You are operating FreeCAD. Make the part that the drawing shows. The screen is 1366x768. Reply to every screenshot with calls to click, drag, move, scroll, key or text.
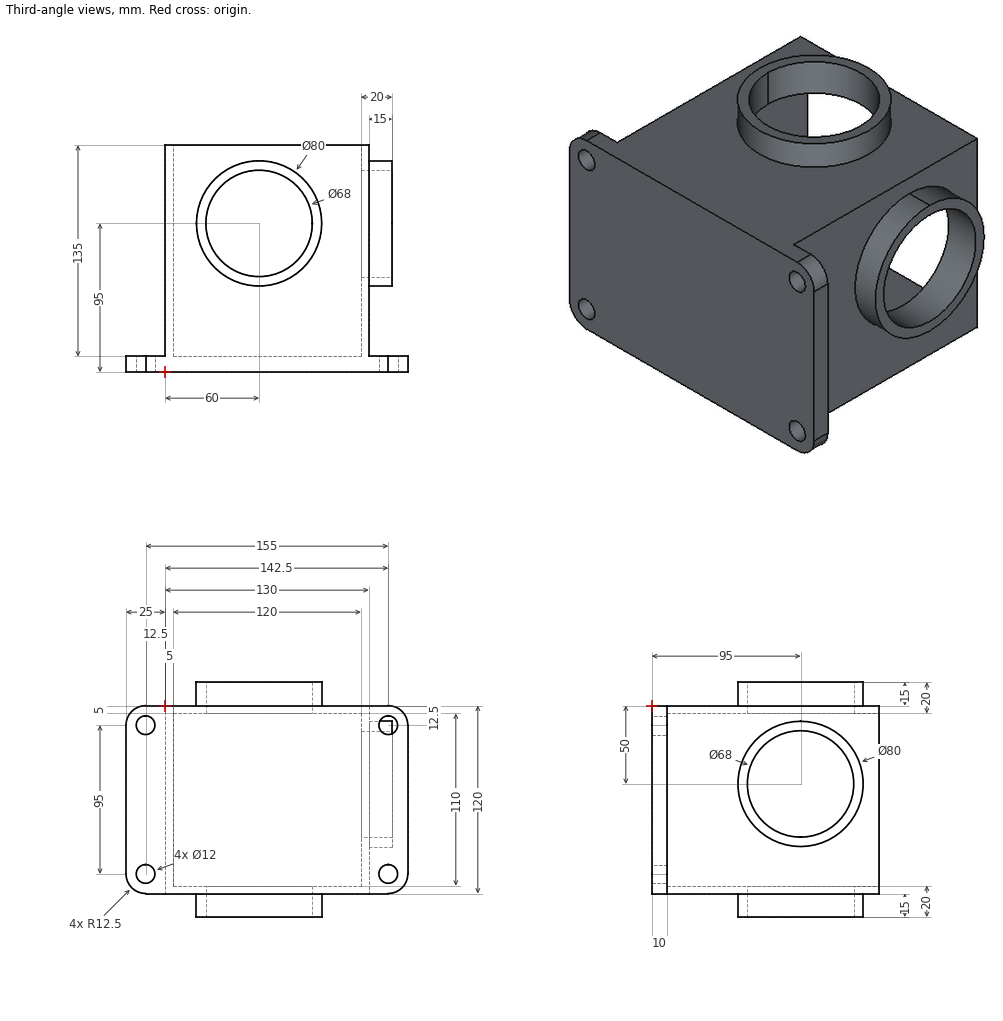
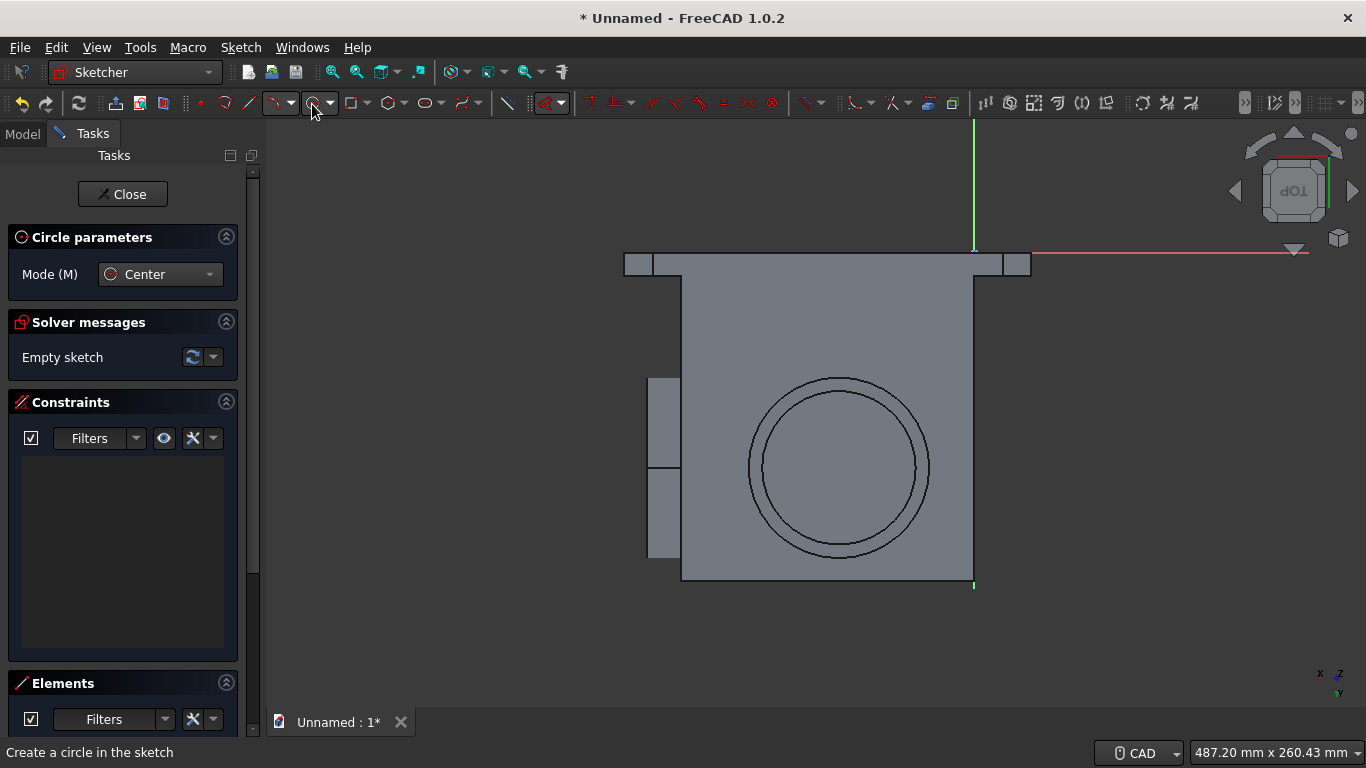
click(839, 468)
move(893, 414)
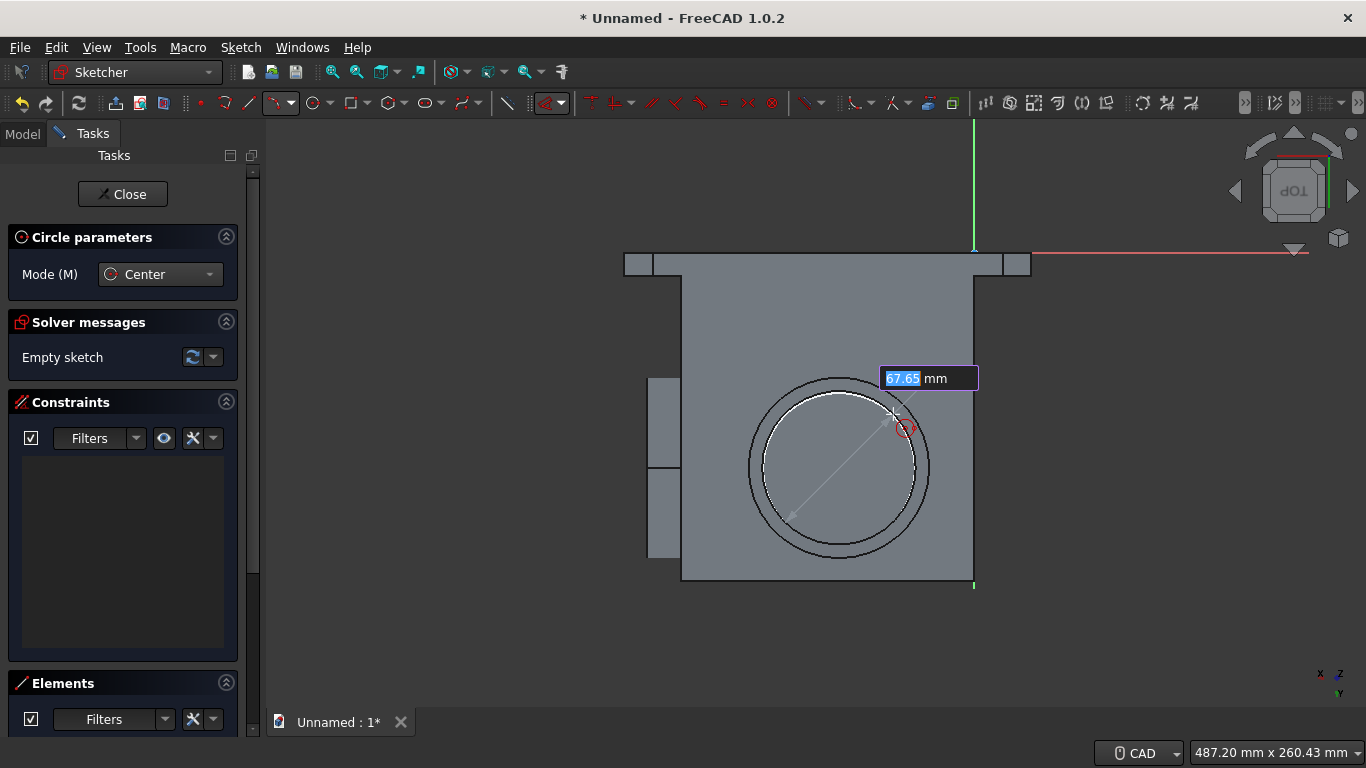
text(68)
key(Return)
key(Escape)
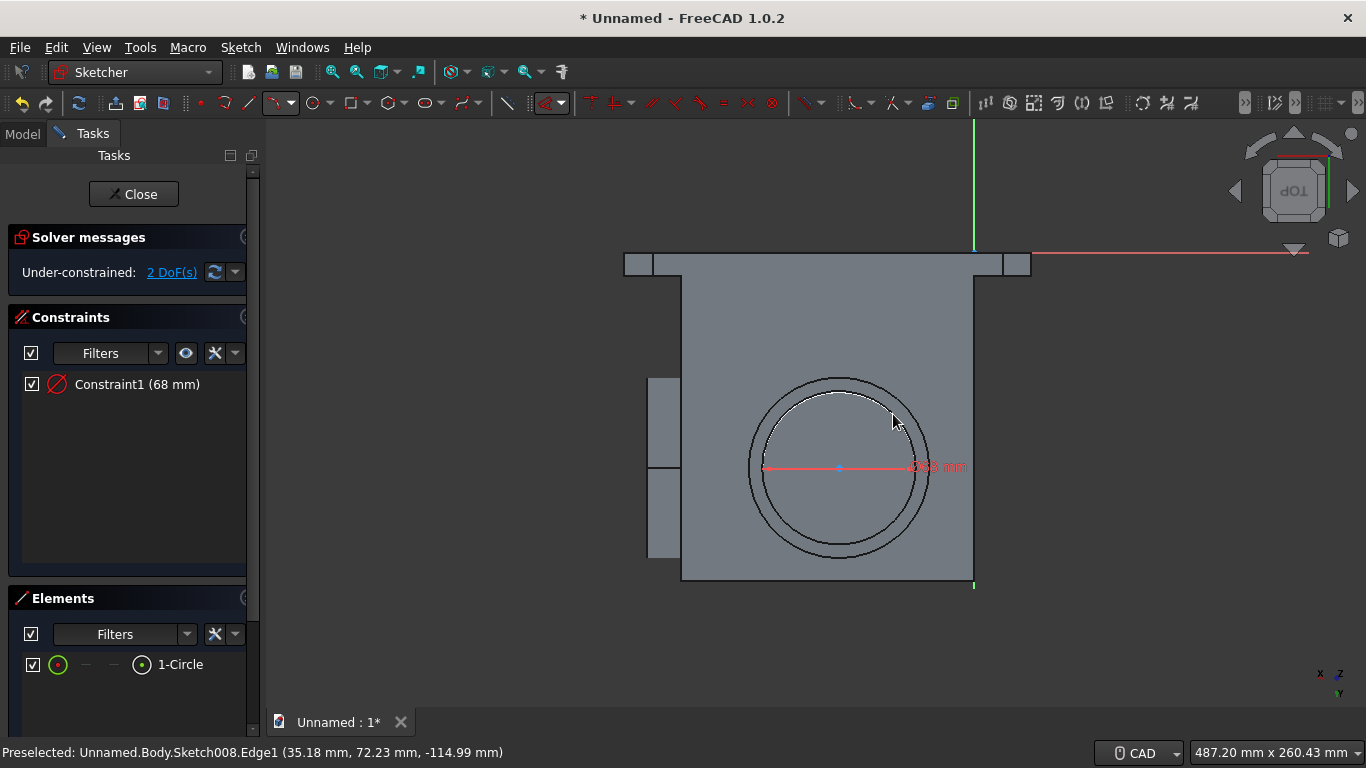
click(839, 469)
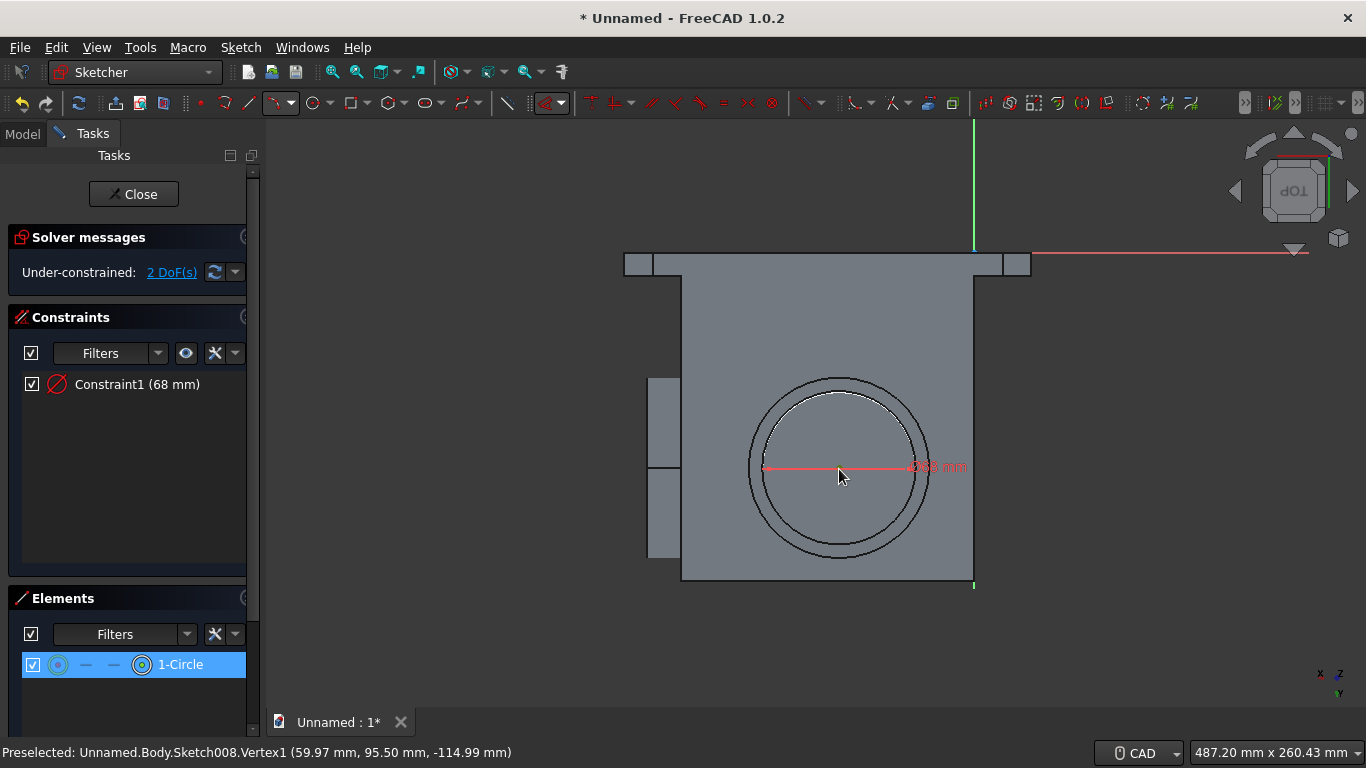
key(l)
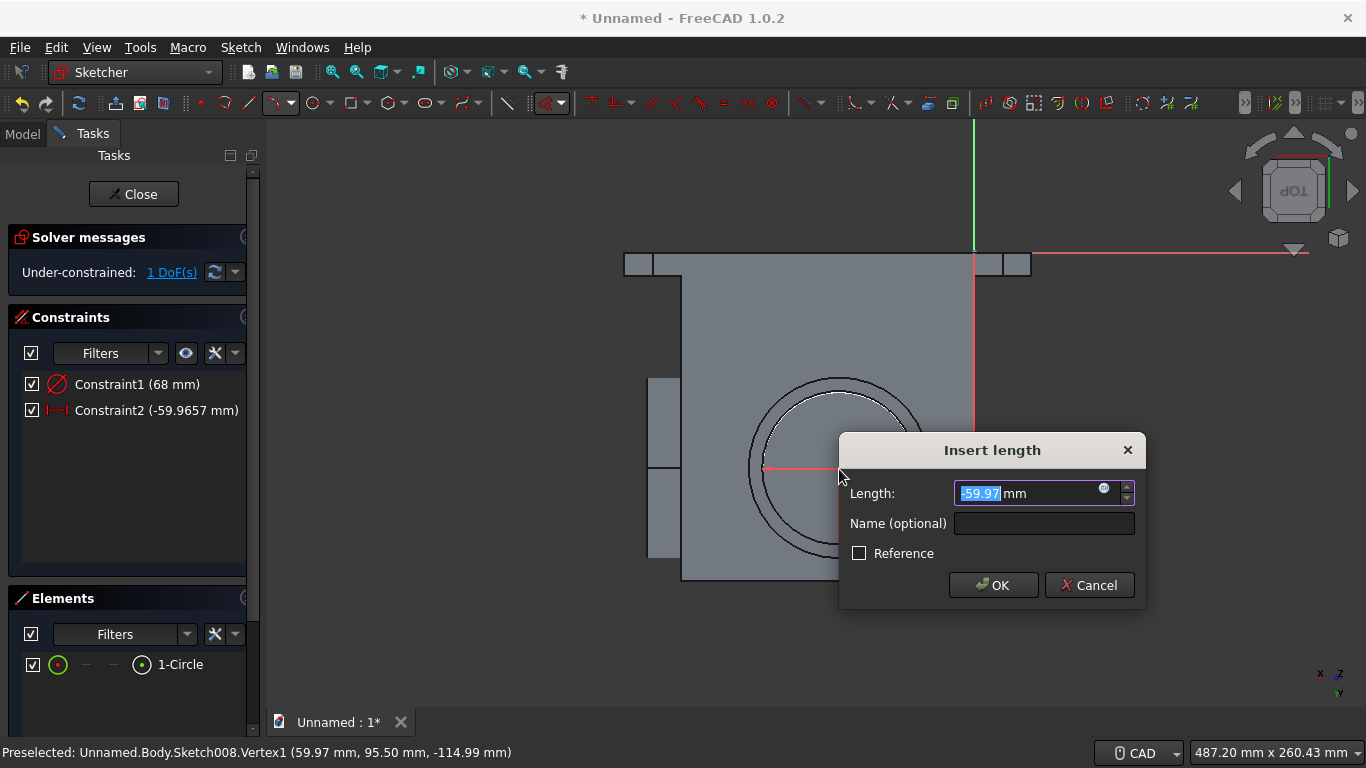
text(-60)
key(Return)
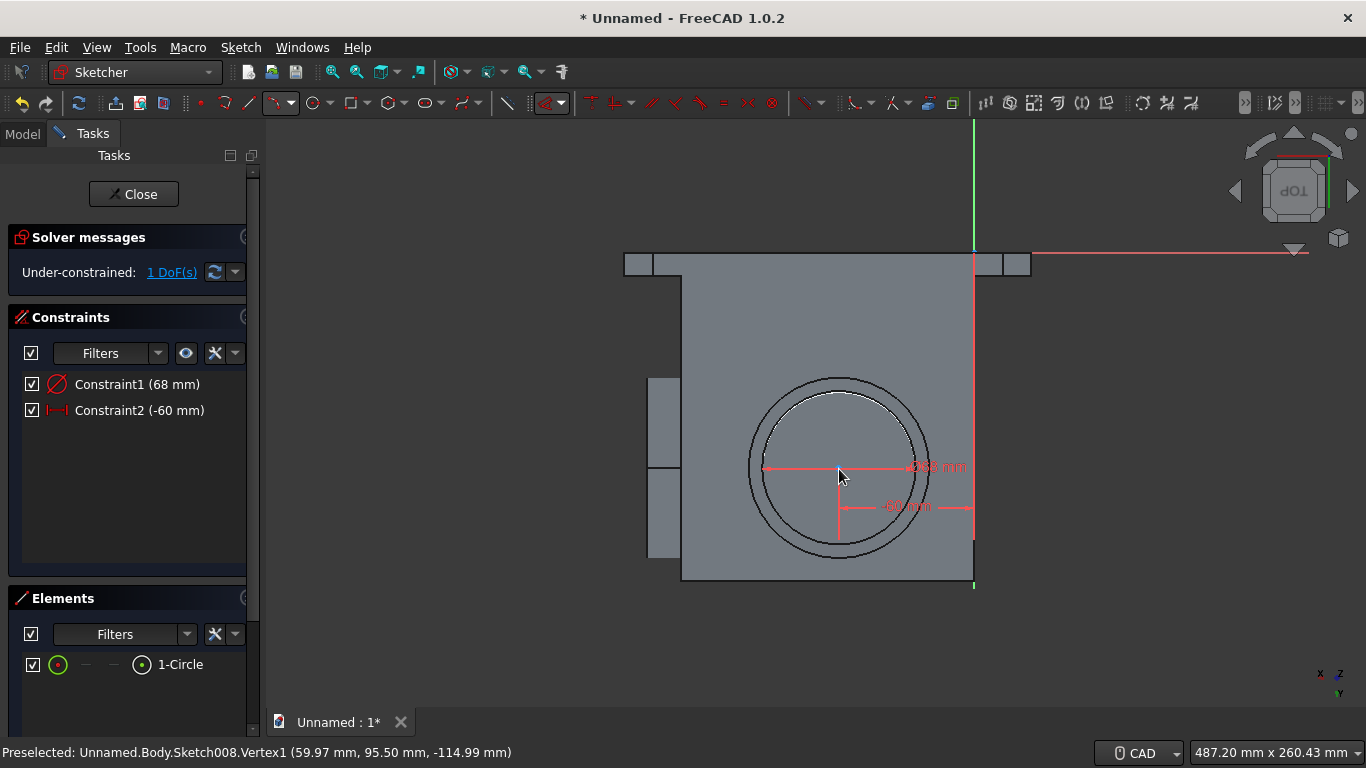
click(839, 469)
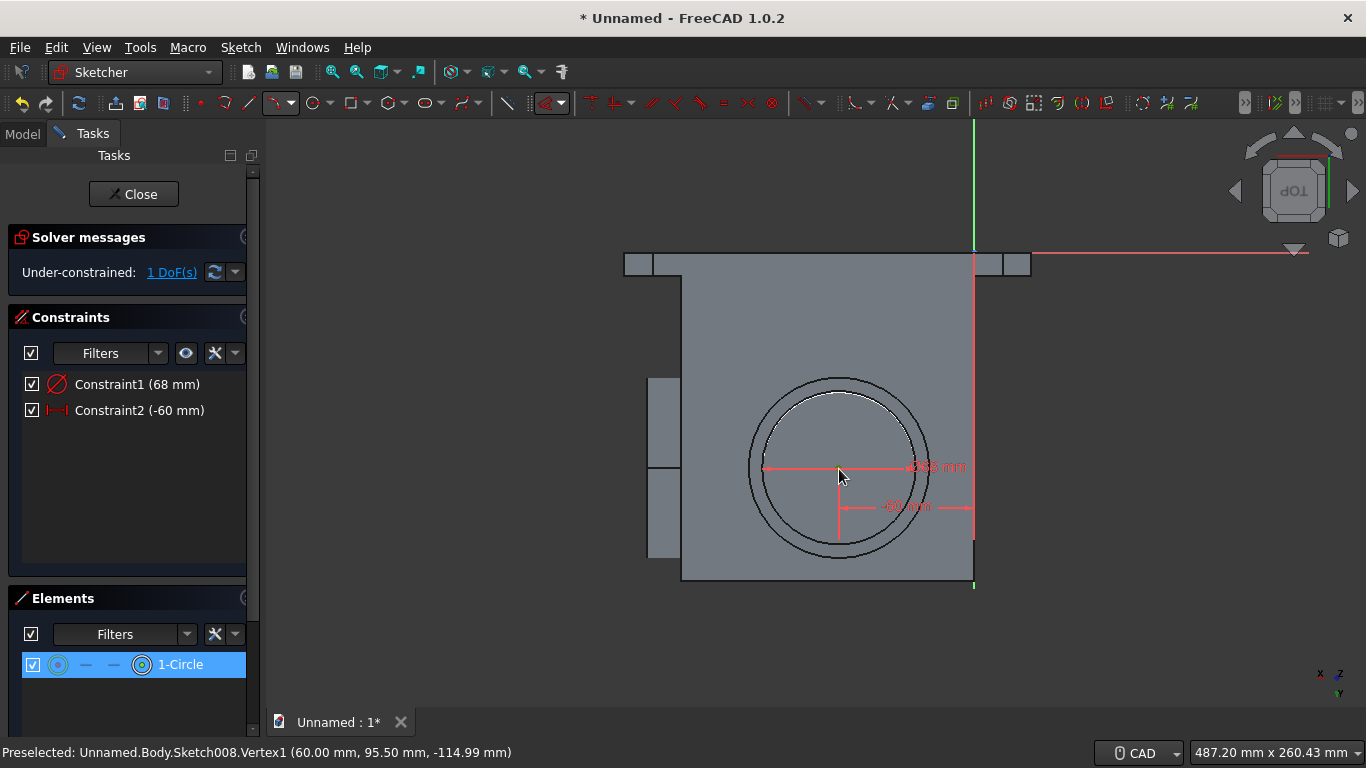
click(564, 104)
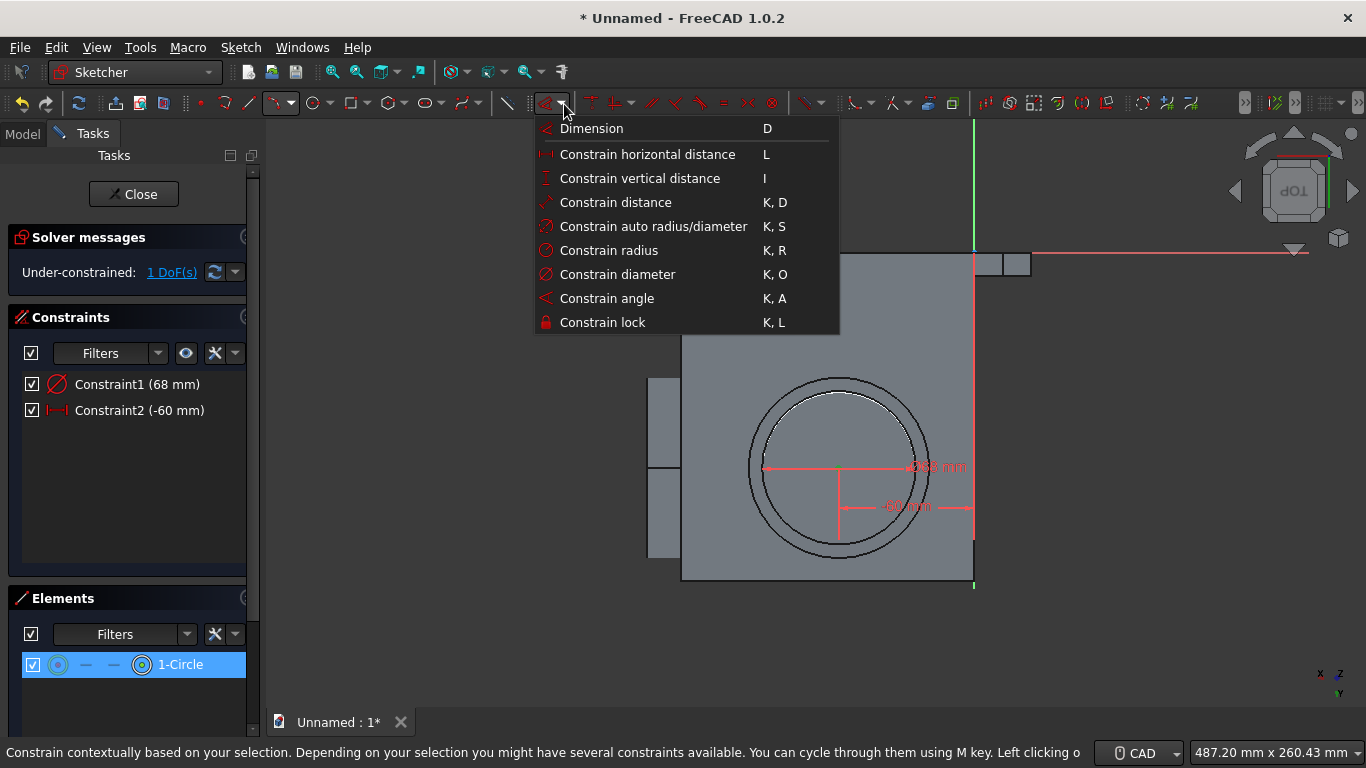
click(687, 178)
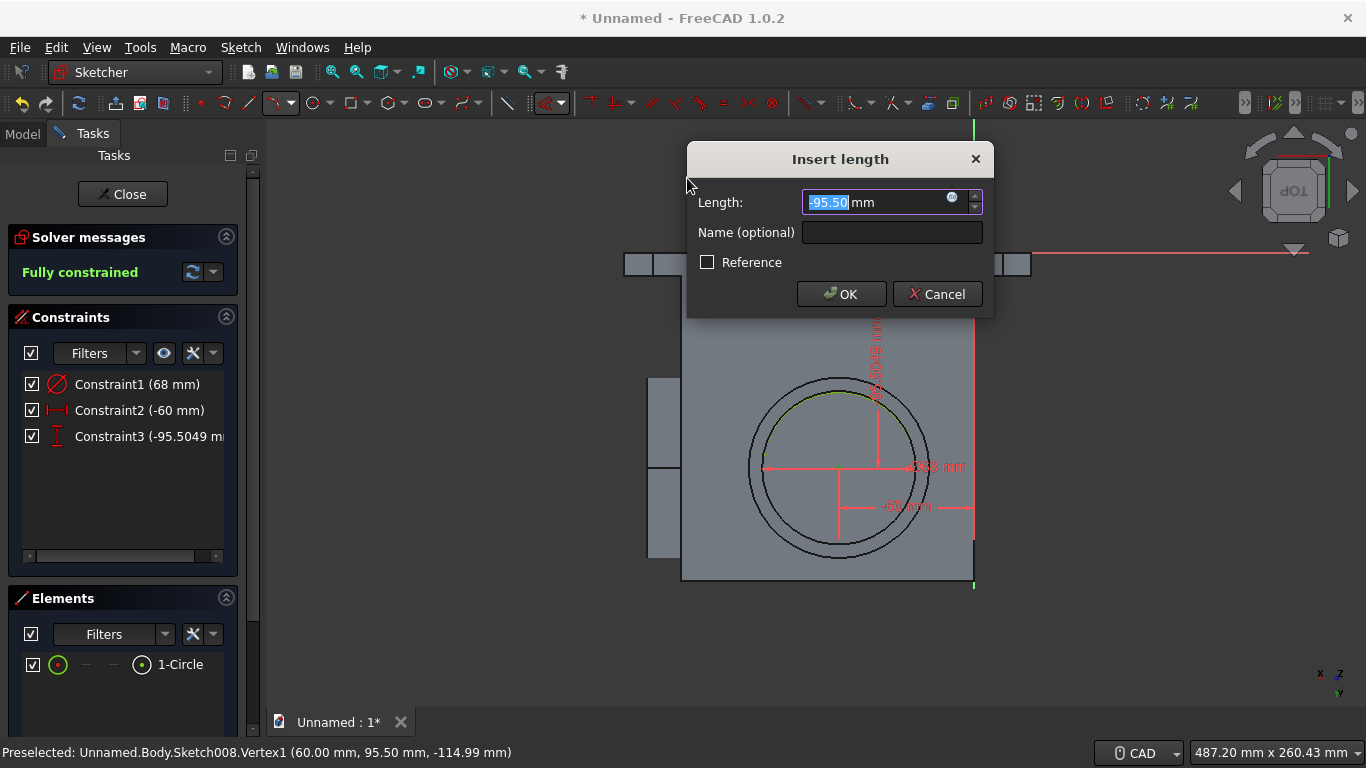
text(-95)
key(Return)